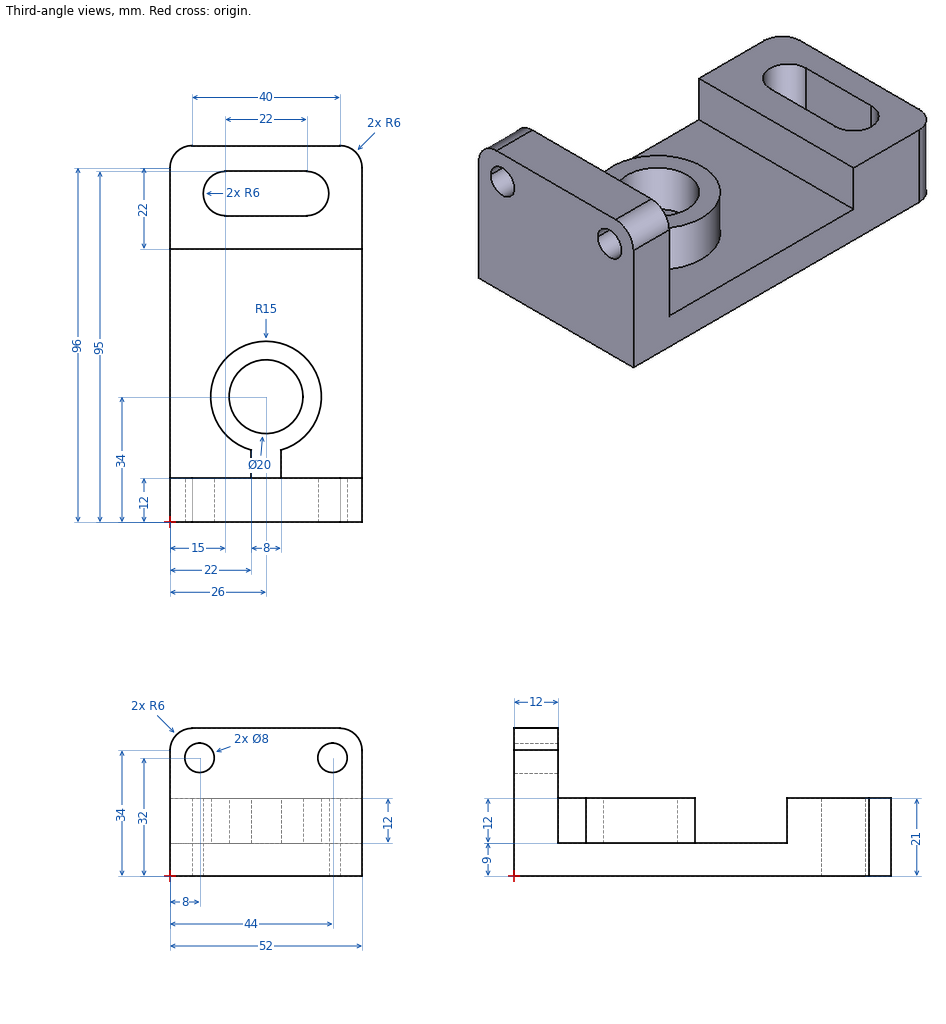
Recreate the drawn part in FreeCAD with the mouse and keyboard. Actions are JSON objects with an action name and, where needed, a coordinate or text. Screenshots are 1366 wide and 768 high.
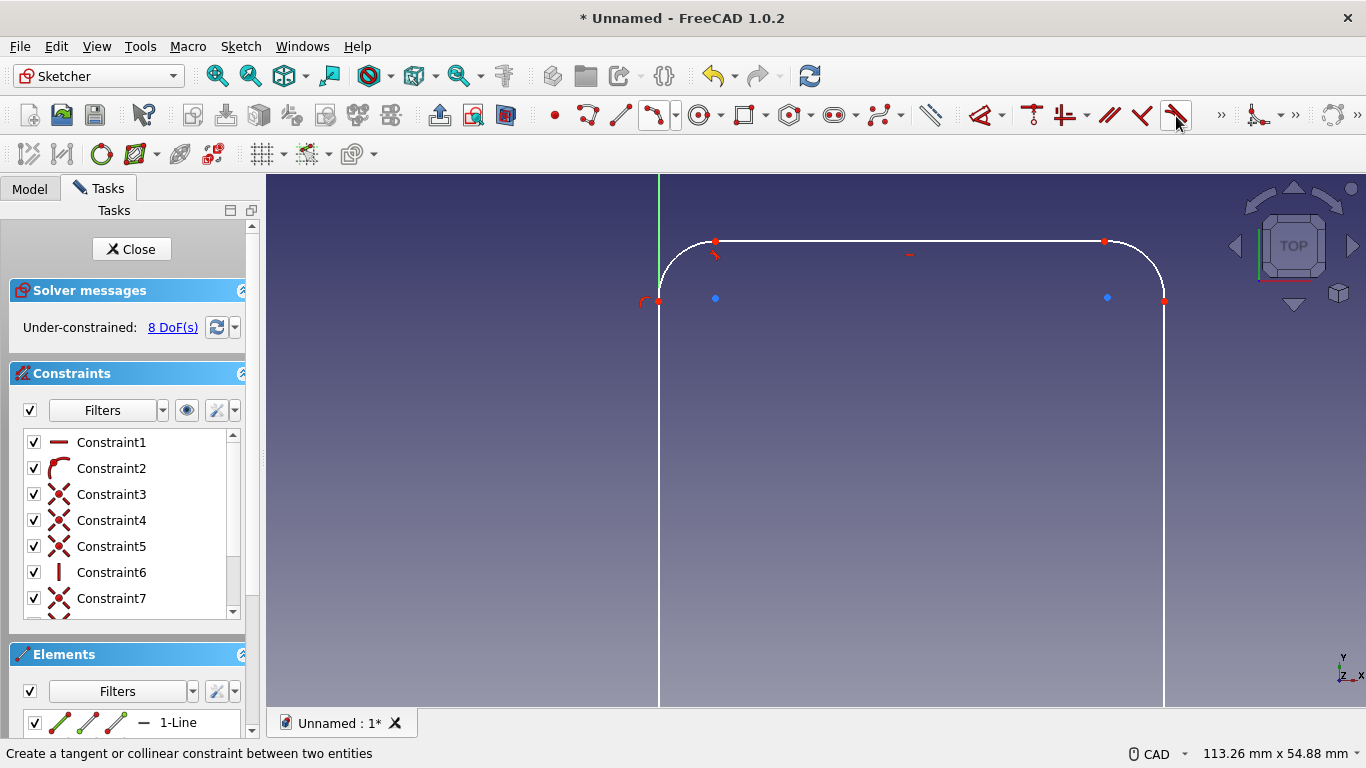
{"action": "left_click", "coordinate": [988, 241]}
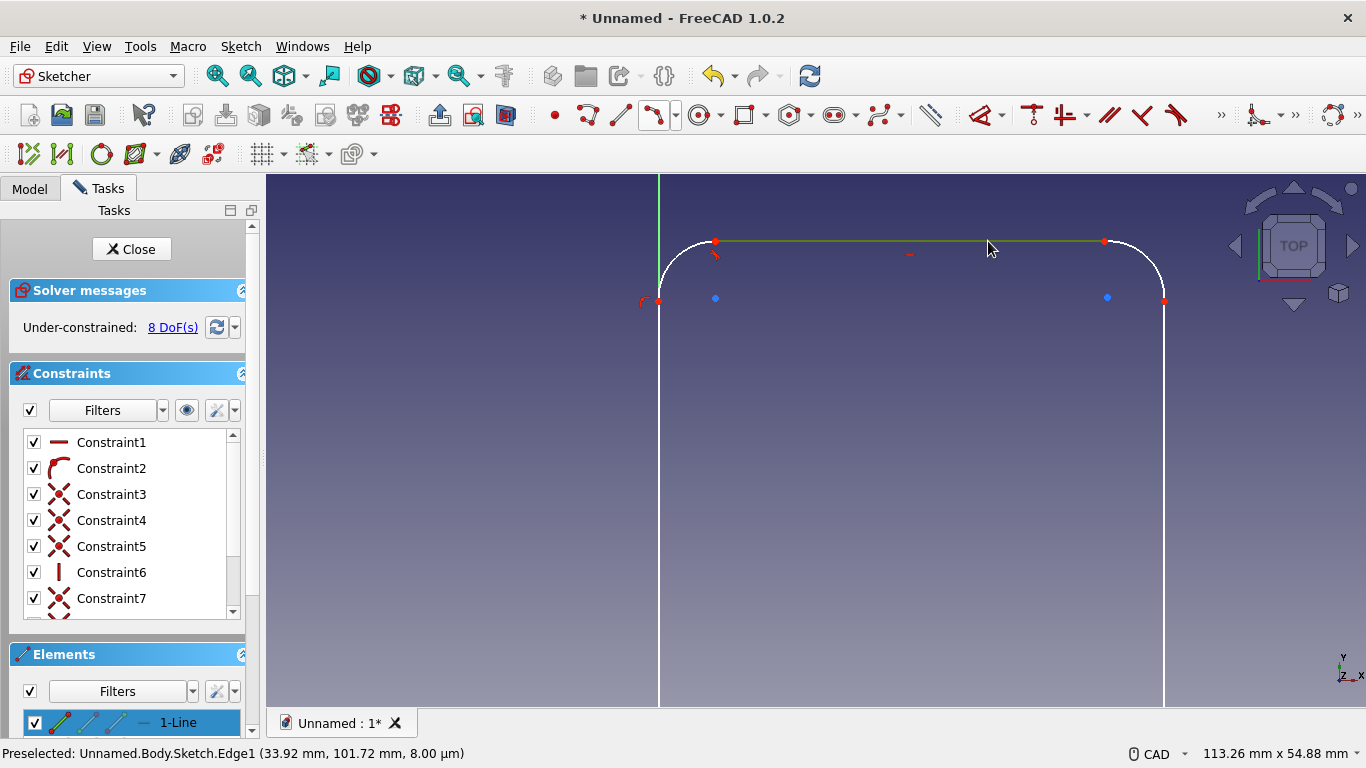
{"action": "left_click", "coordinate": [1159, 273]}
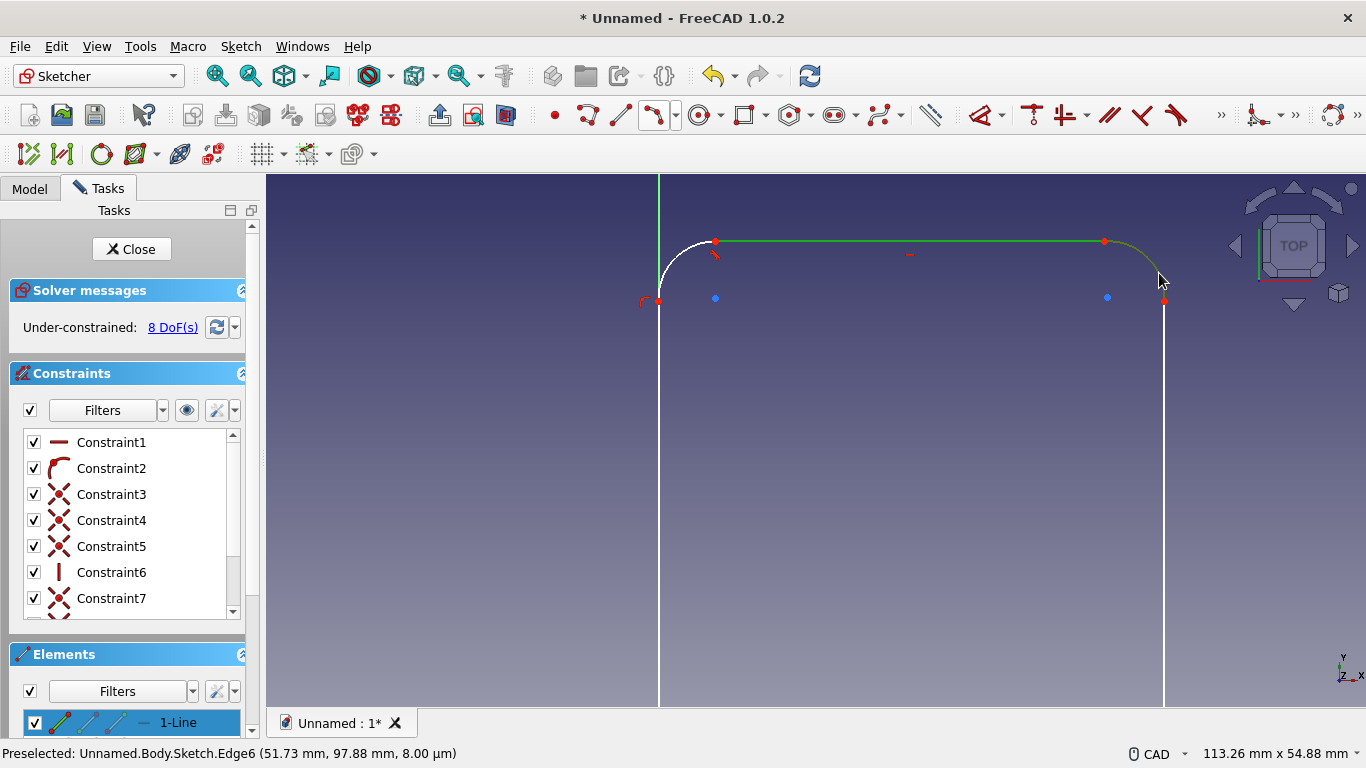
{"action": "left_click", "coordinate": [1176, 116]}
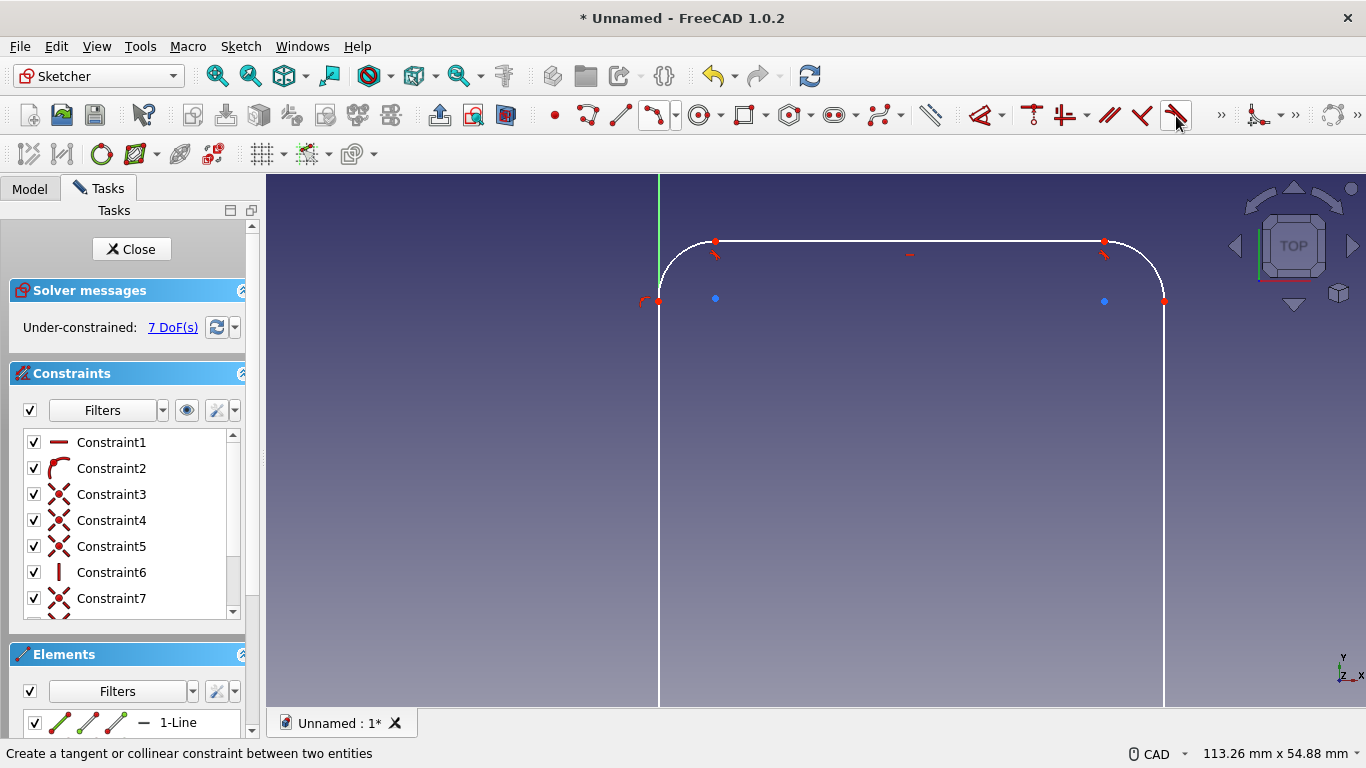
{"action": "left_click", "coordinate": [659, 580]}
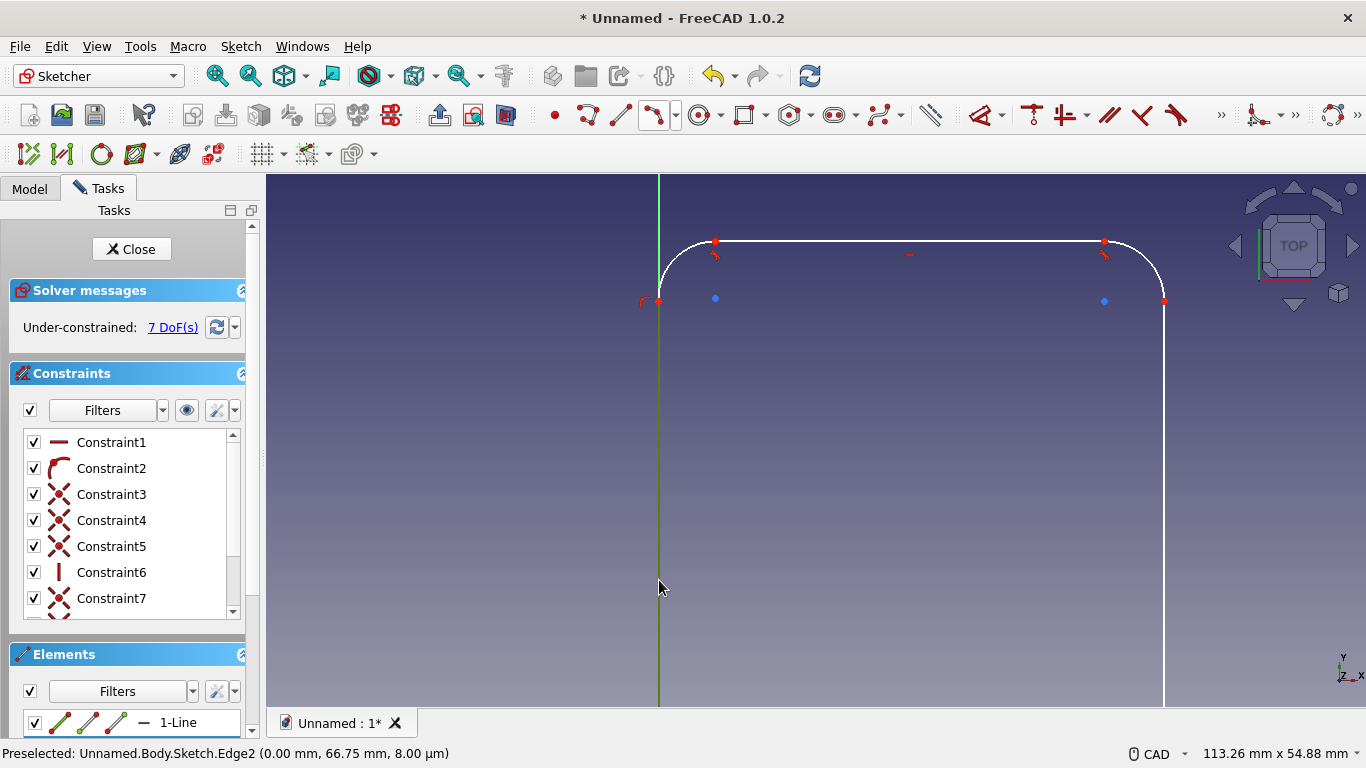
{"action": "left_click", "coordinate": [689, 248]}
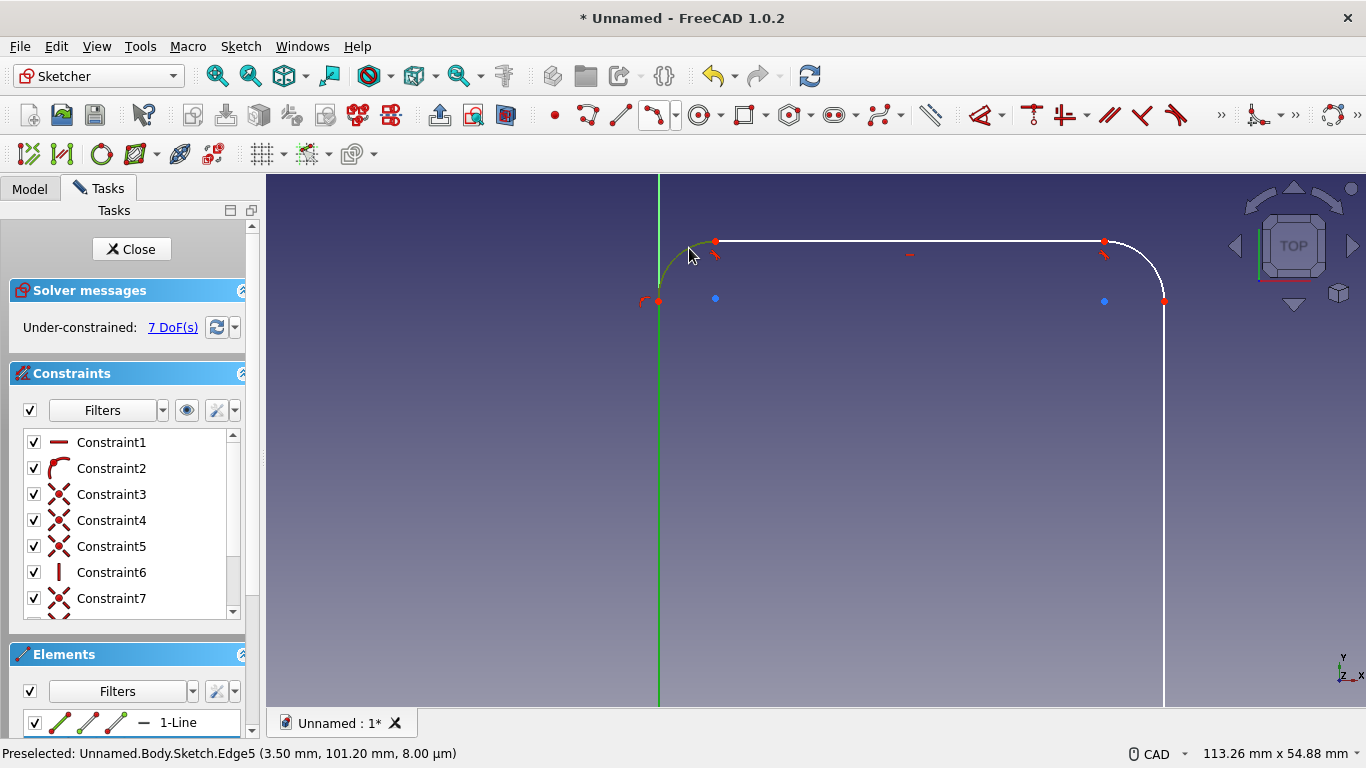
{"action": "left_click", "coordinate": [1176, 116]}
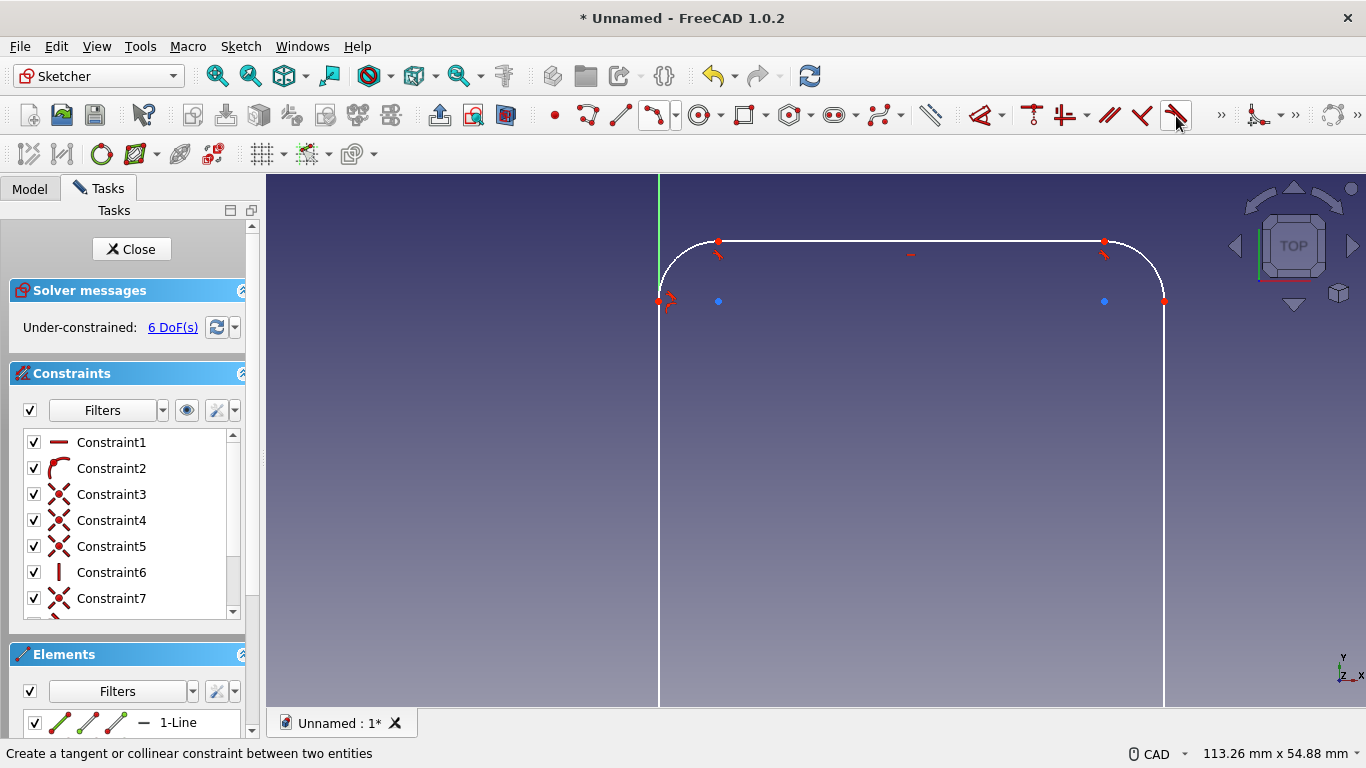
{"action": "left_click", "coordinate": [1164, 572]}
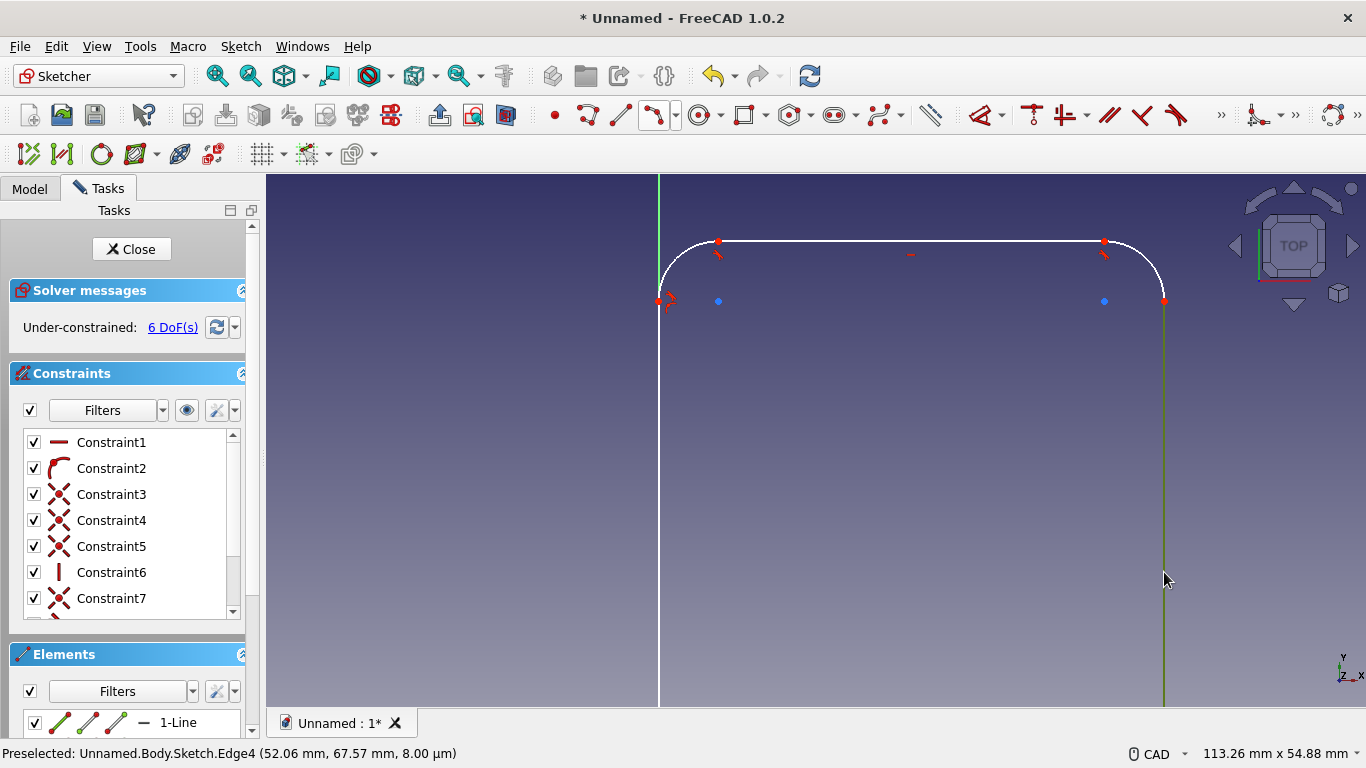
{"action": "left_click", "coordinate": [1158, 274]}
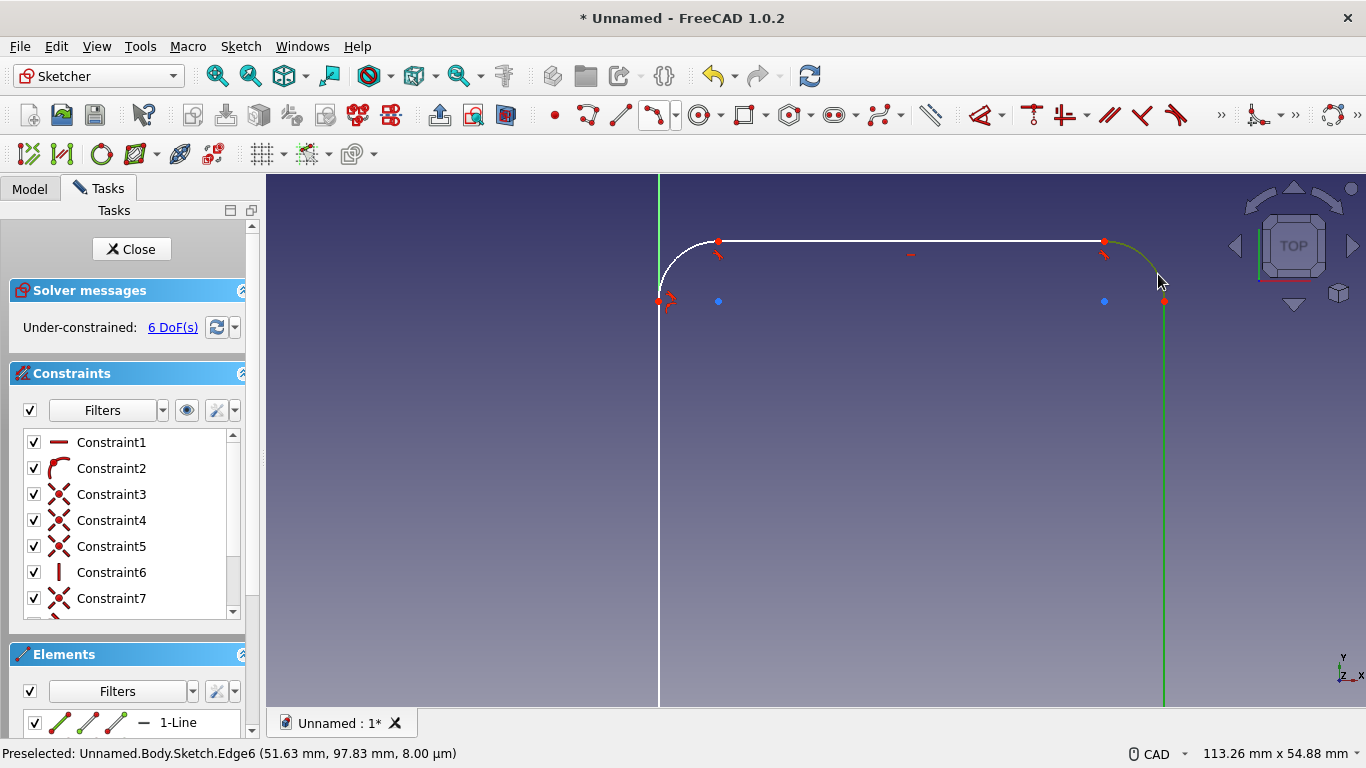
{"action": "left_click", "coordinate": [1176, 116]}